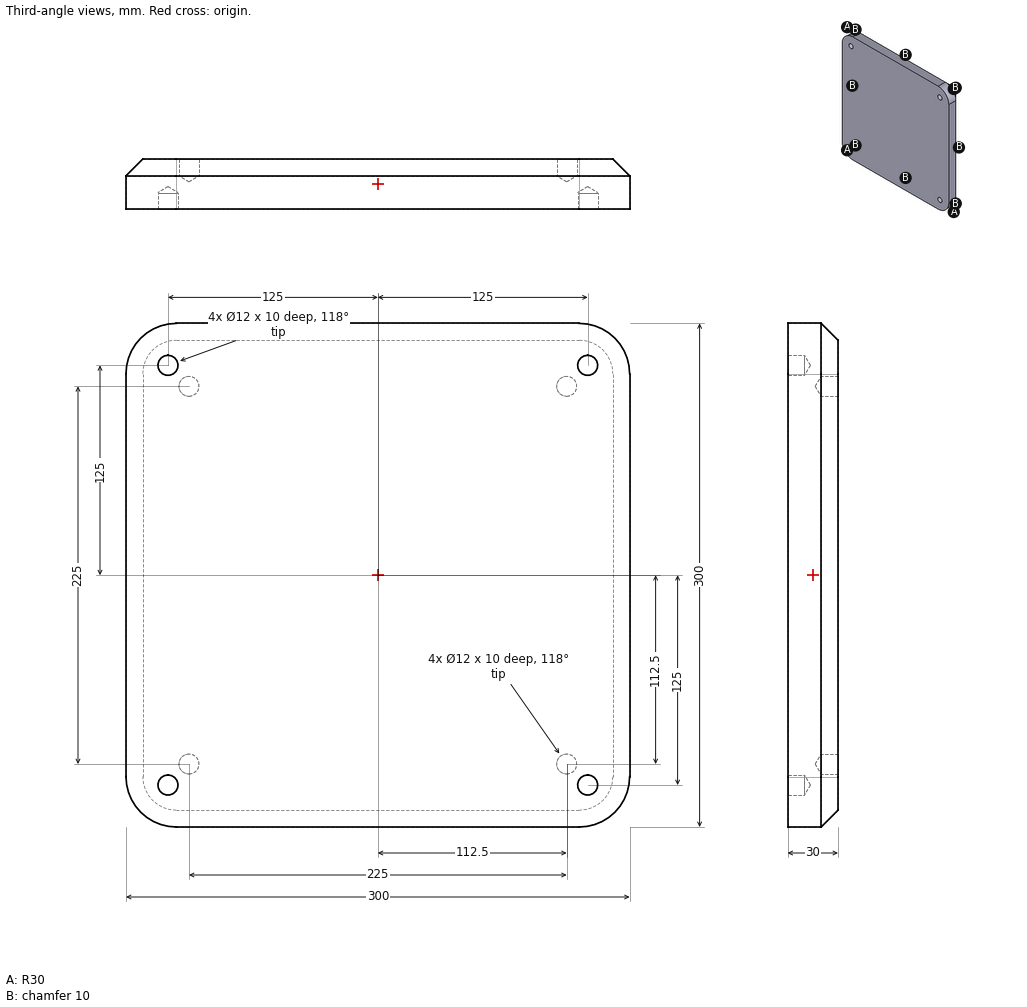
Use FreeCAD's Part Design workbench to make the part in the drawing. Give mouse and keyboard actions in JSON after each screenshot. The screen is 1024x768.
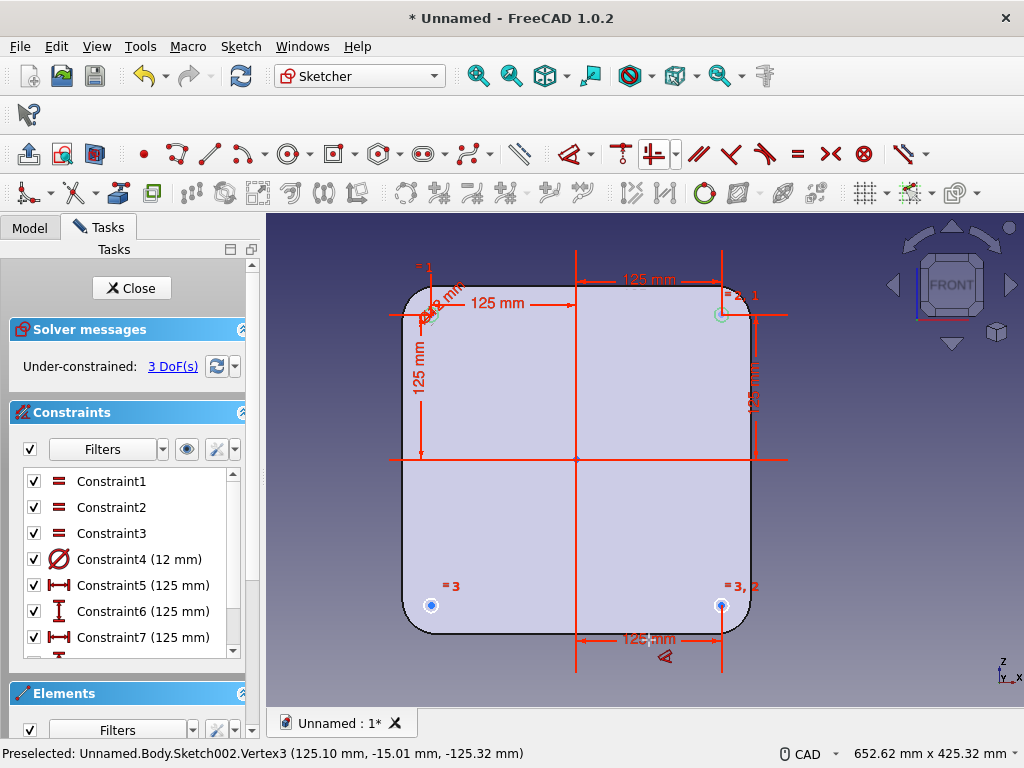
{"action": "left_click", "coordinate": [722, 606]}
{"action": "left_click", "coordinate": [756, 533]}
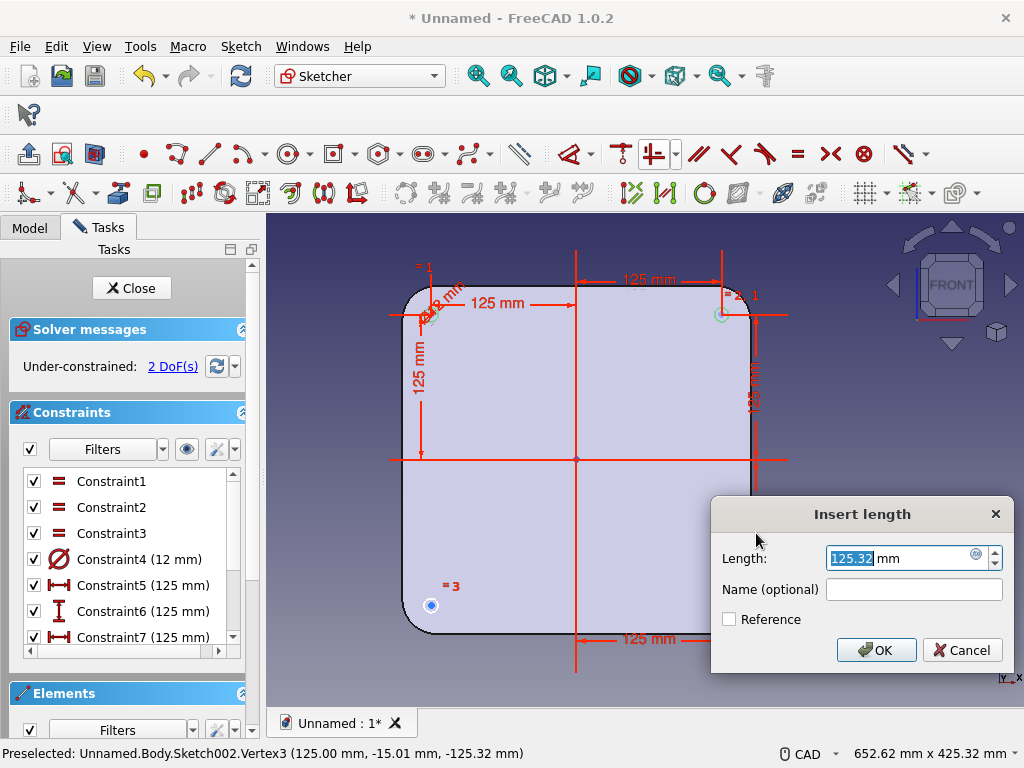
{"action": "type", "text": "125"}
{"action": "key", "text": "Return"}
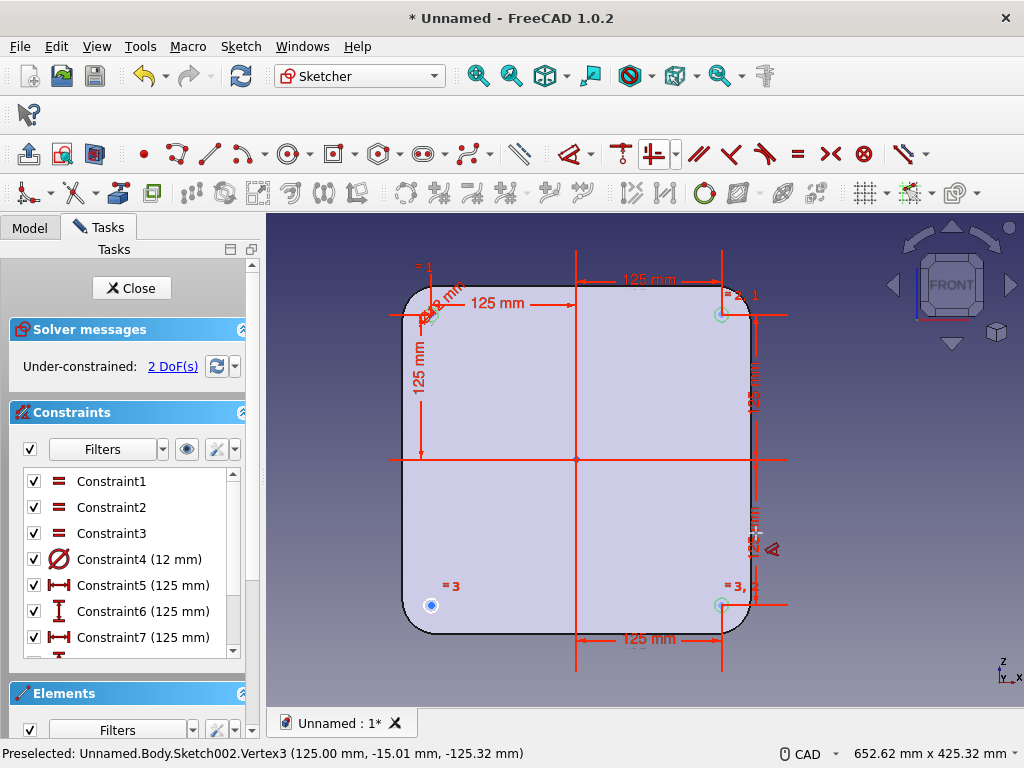
{"action": "left_click", "coordinate": [431, 606]}
{"action": "left_click", "coordinate": [504, 640]}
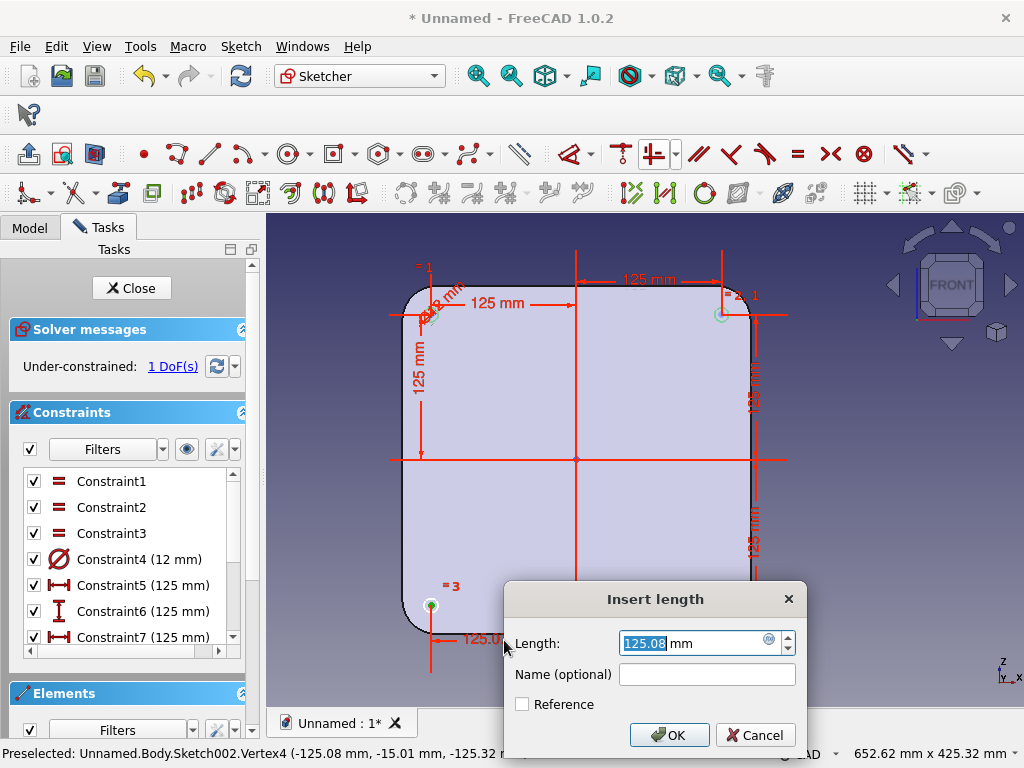
{"action": "type", "text": "125"}
{"action": "key", "text": "Return"}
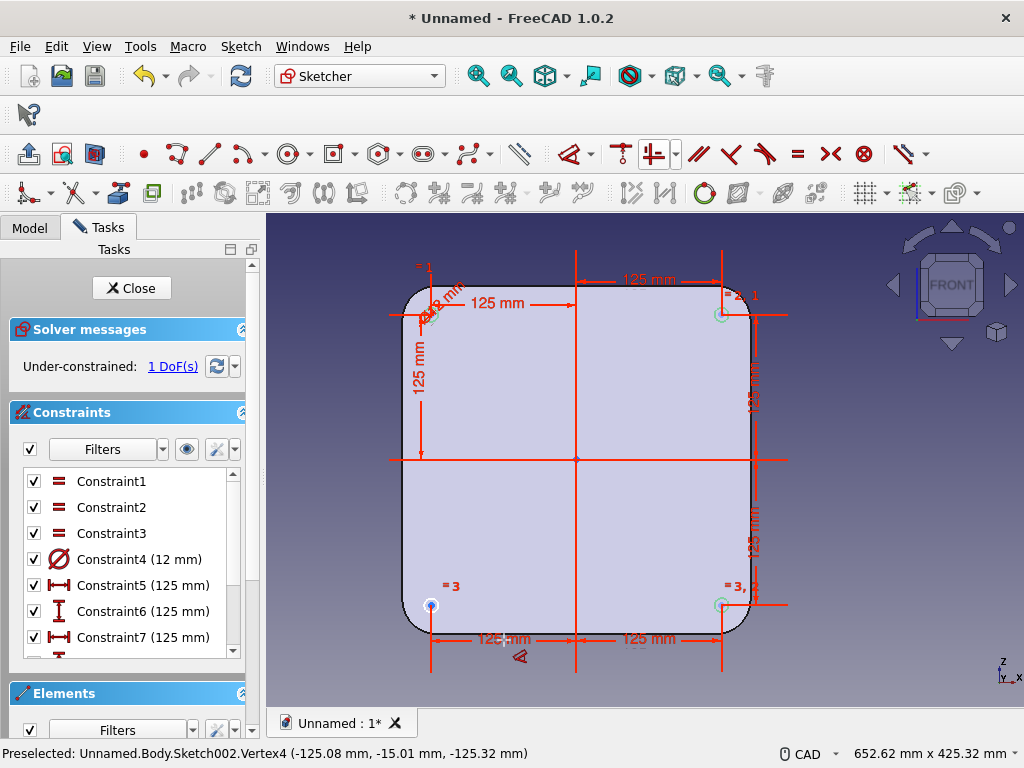
{"action": "left_click", "coordinate": [431, 606]}
{"action": "left_click", "coordinate": [397, 533]}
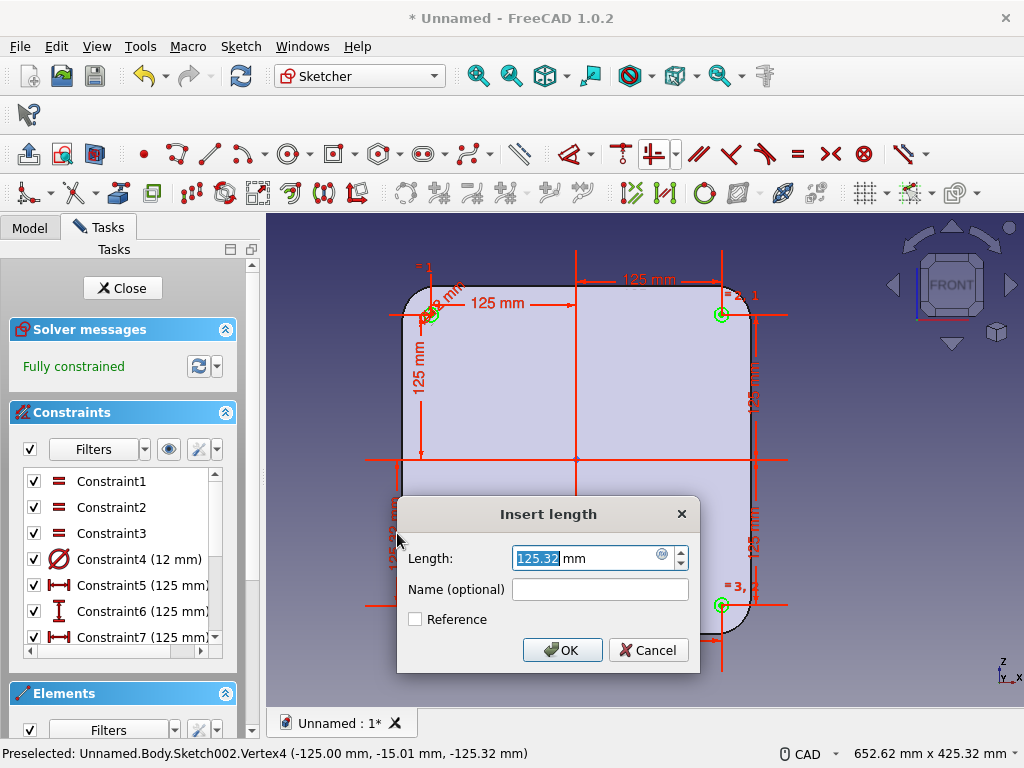
{"action": "type", "text": "125"}
{"action": "key", "text": "Return"}
{"action": "key", "text": "Escape"}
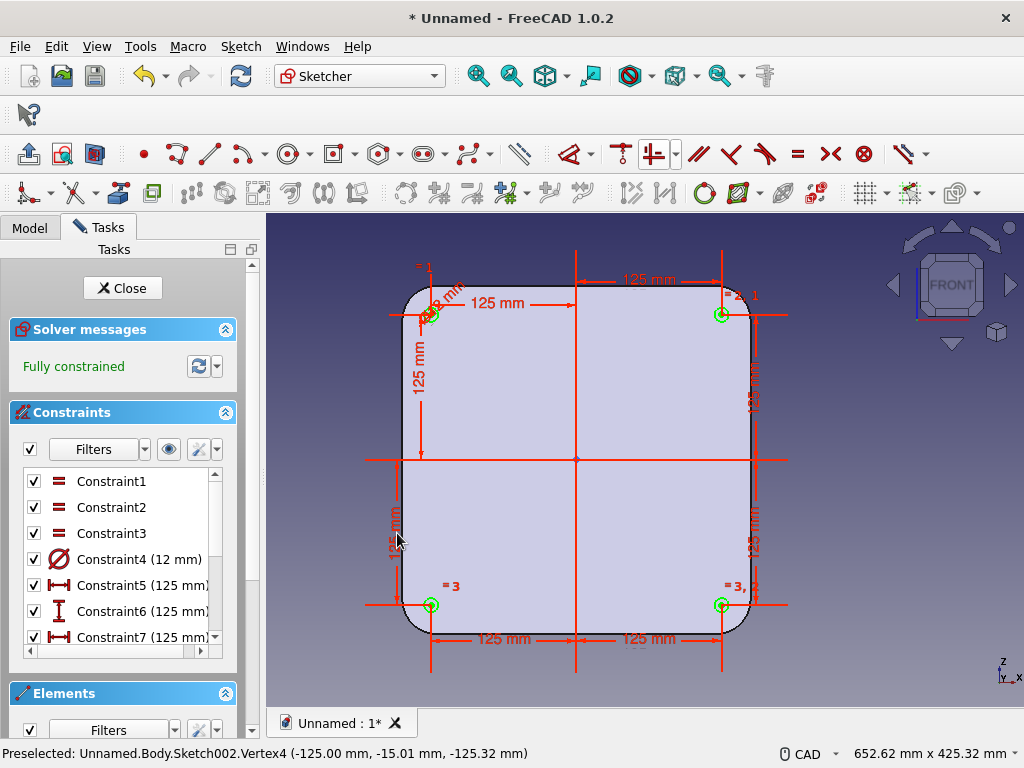
{"action": "left_click", "coordinate": [123, 288]}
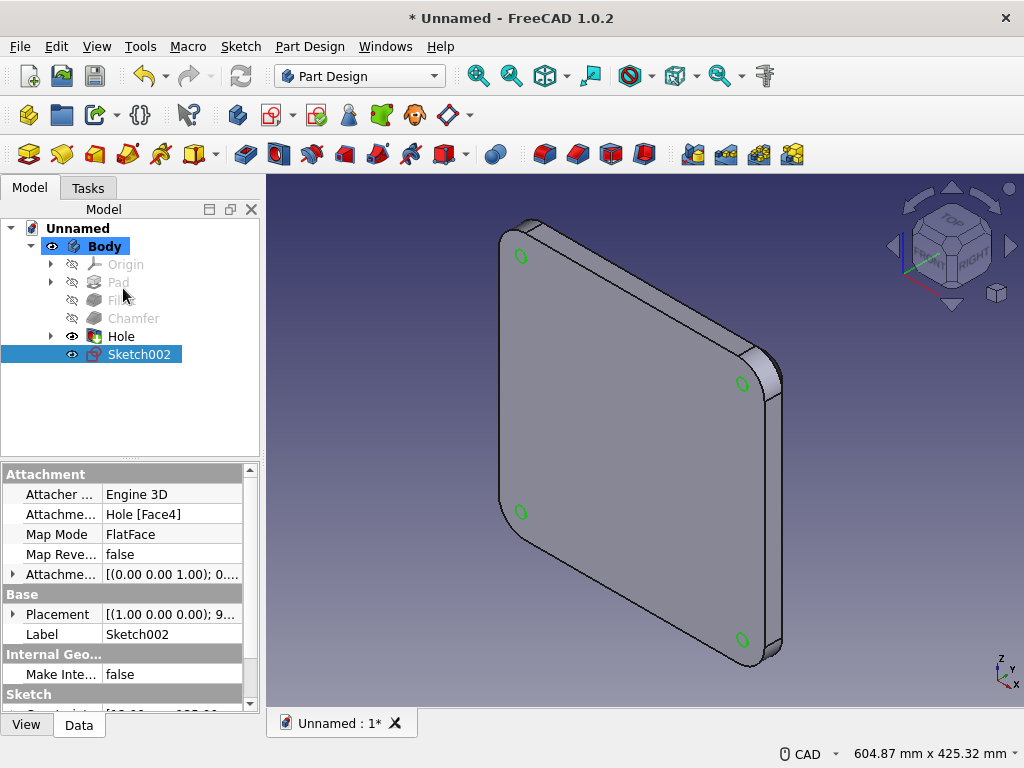
{"action": "left_click", "coordinate": [279, 154]}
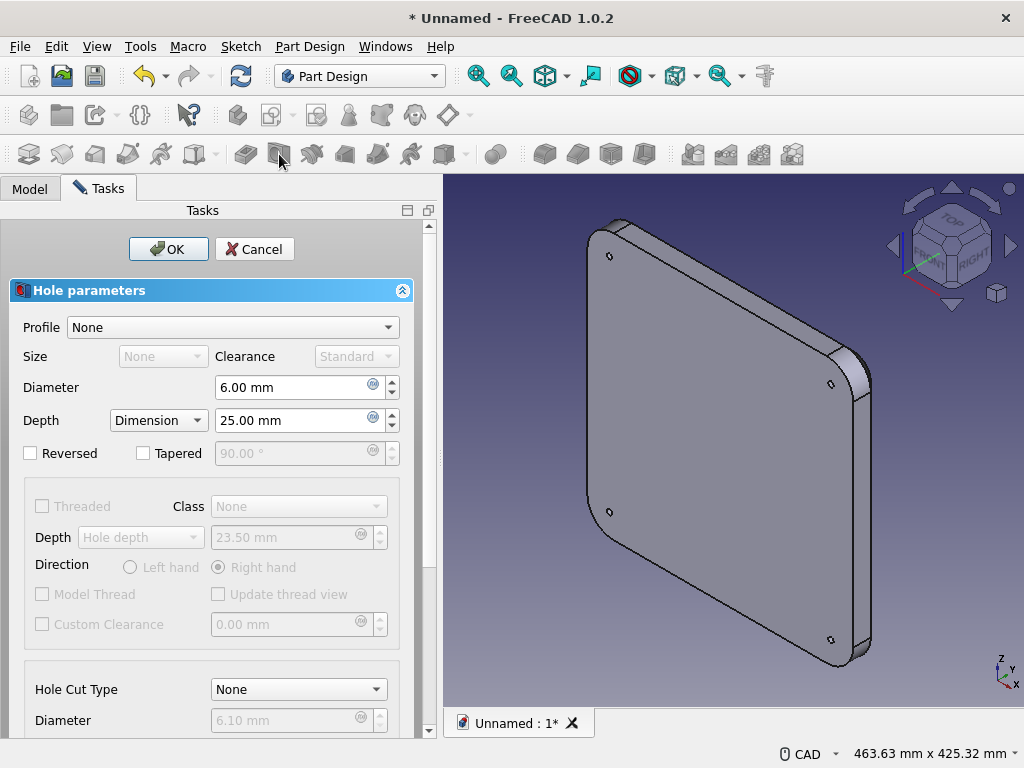
{"action": "triple_click", "coordinate": [300, 388]}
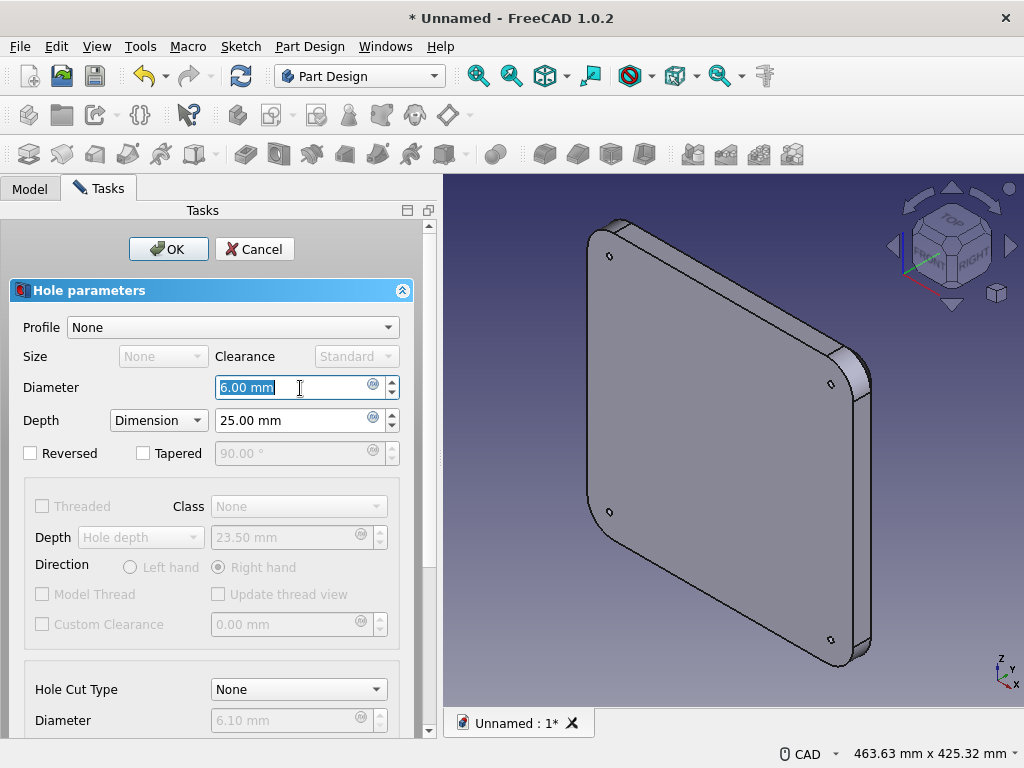
{"action": "type", "text": "12"}
{"action": "key", "text": "Tab"}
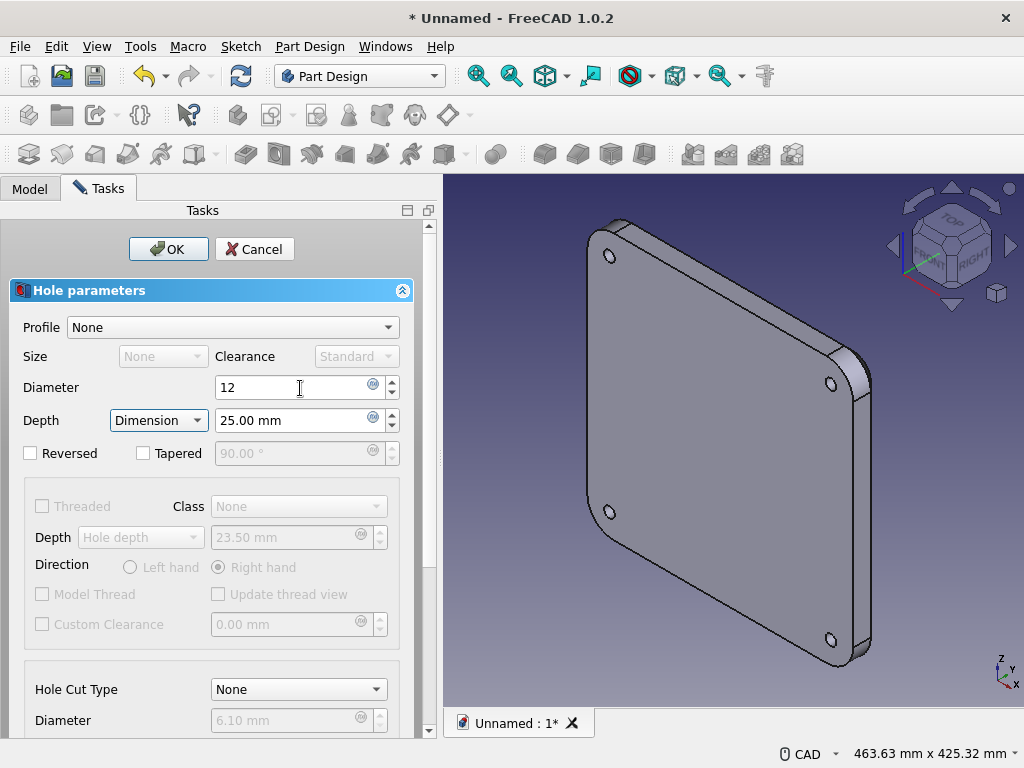
{"action": "triple_click", "coordinate": [300, 420]}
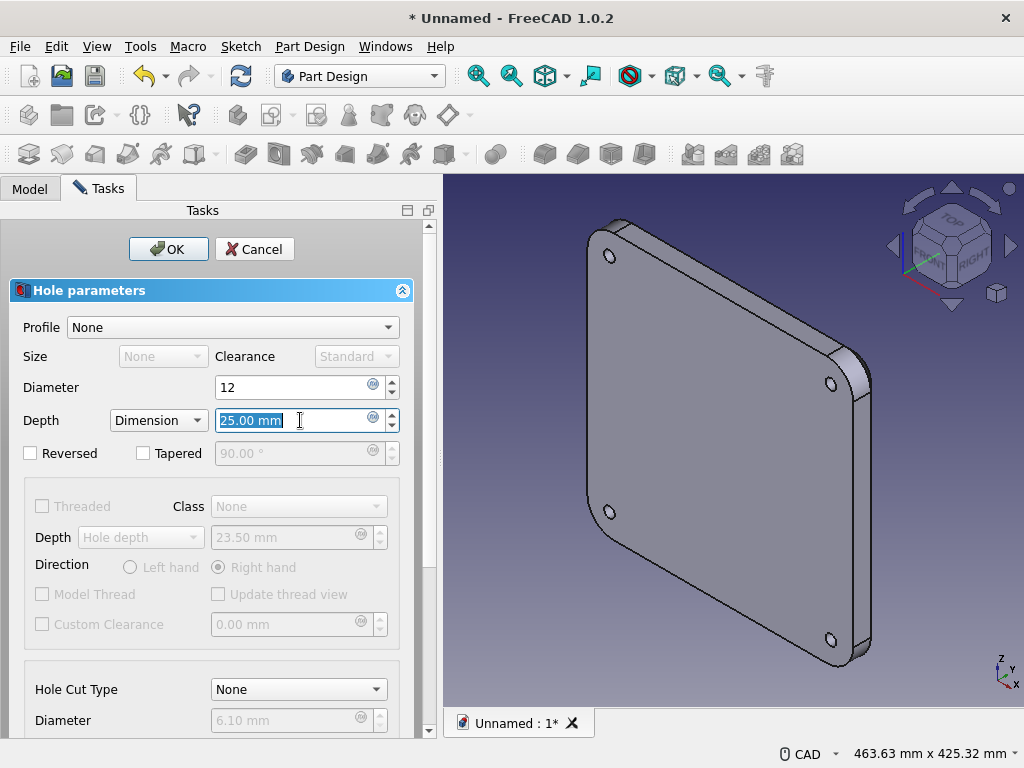
{"action": "type", "text": "10"}
{"action": "key", "text": "Tab"}